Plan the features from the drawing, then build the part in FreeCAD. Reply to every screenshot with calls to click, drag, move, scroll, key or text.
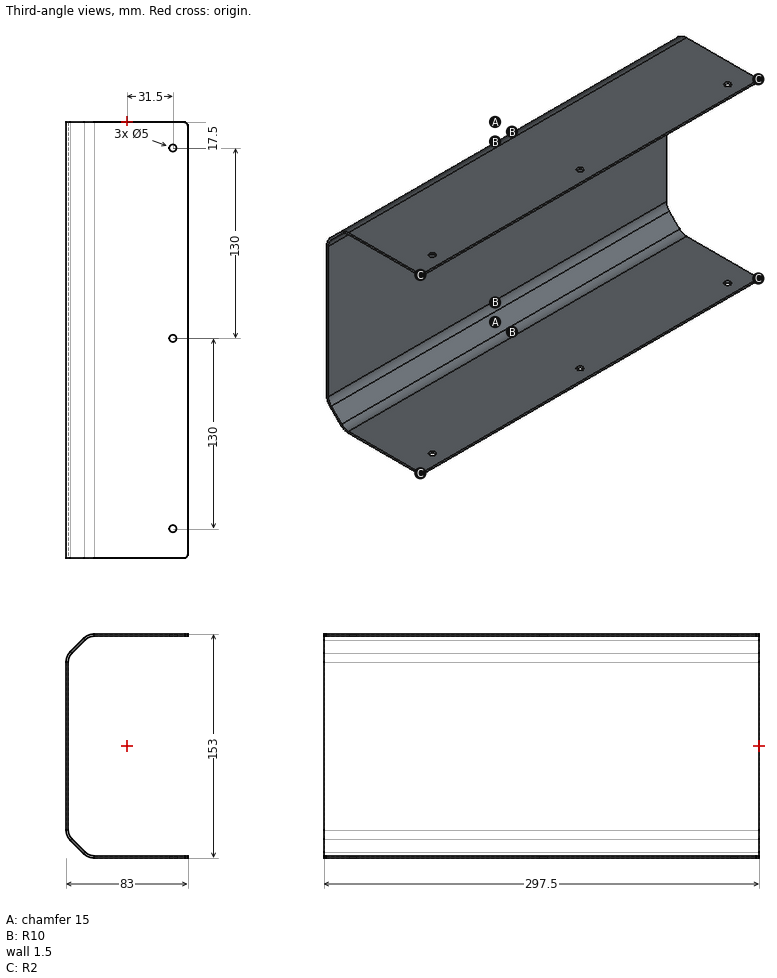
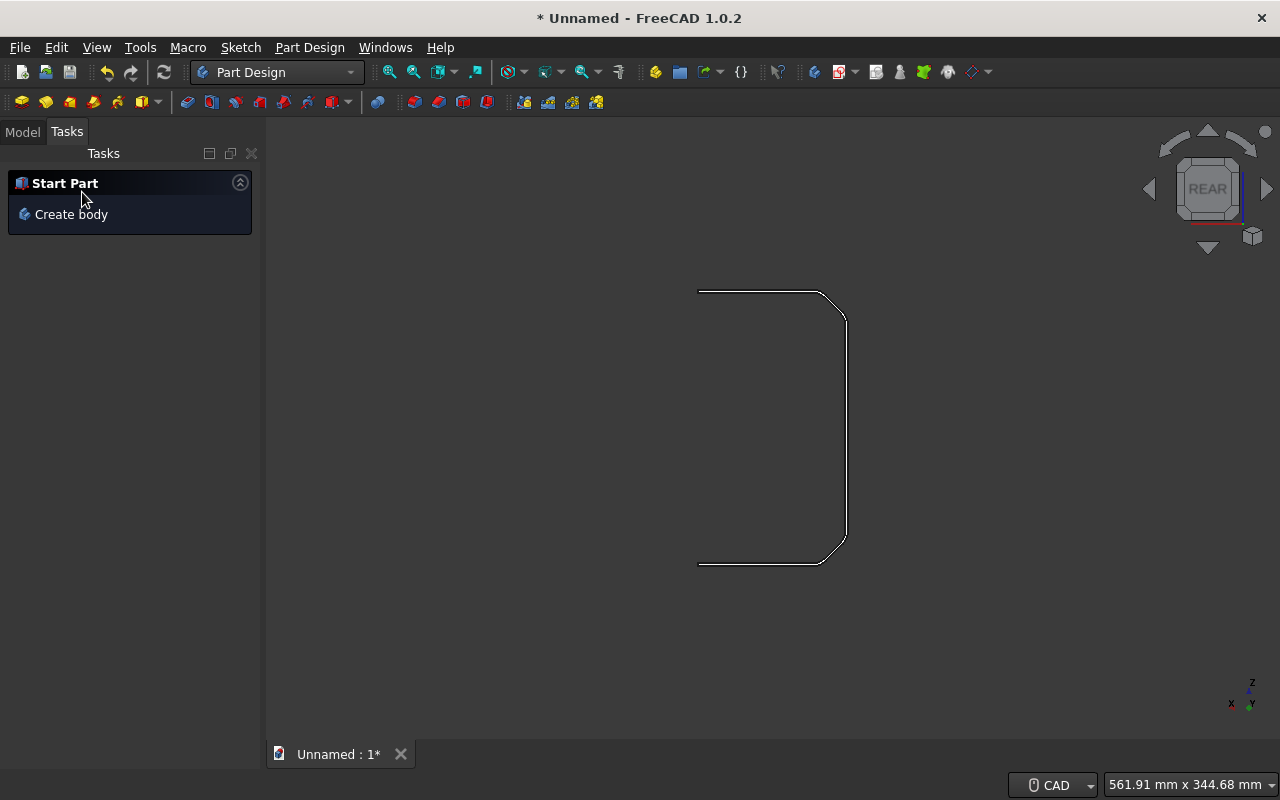
click(390, 72)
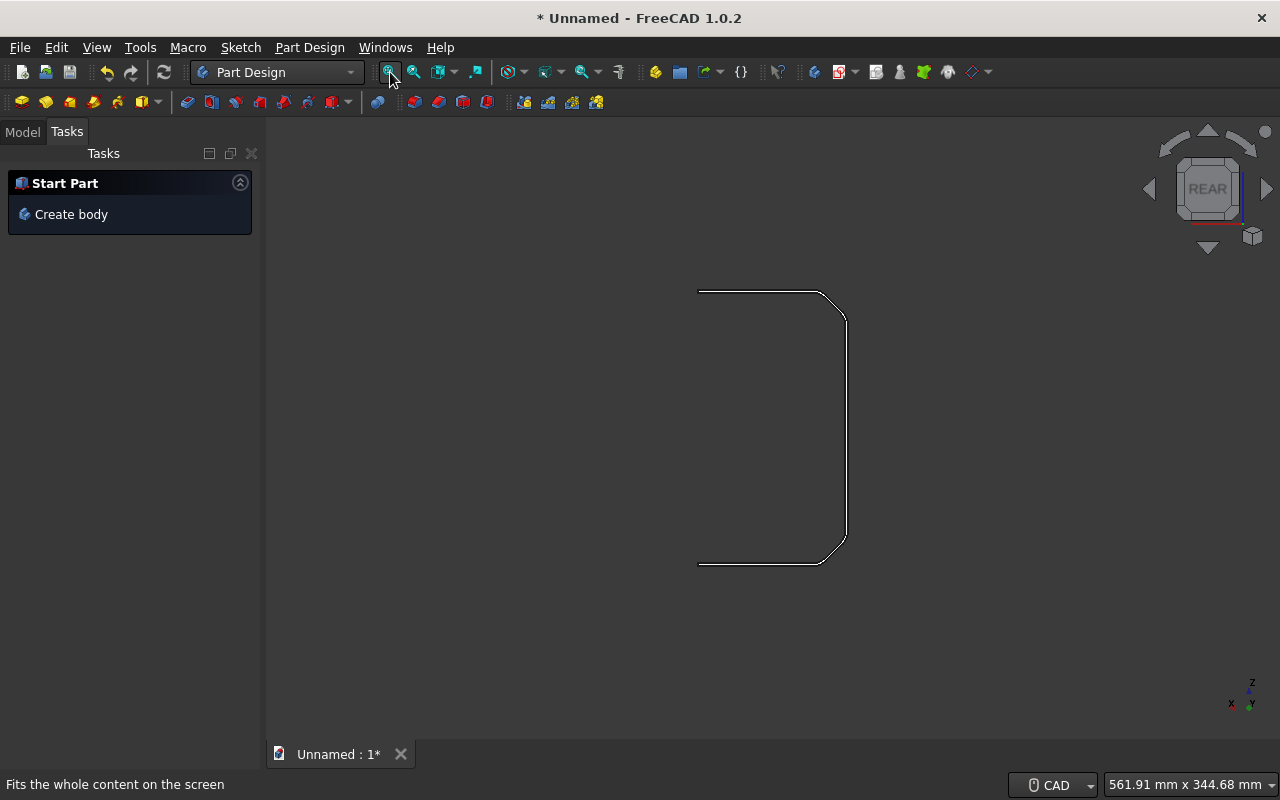
key(0)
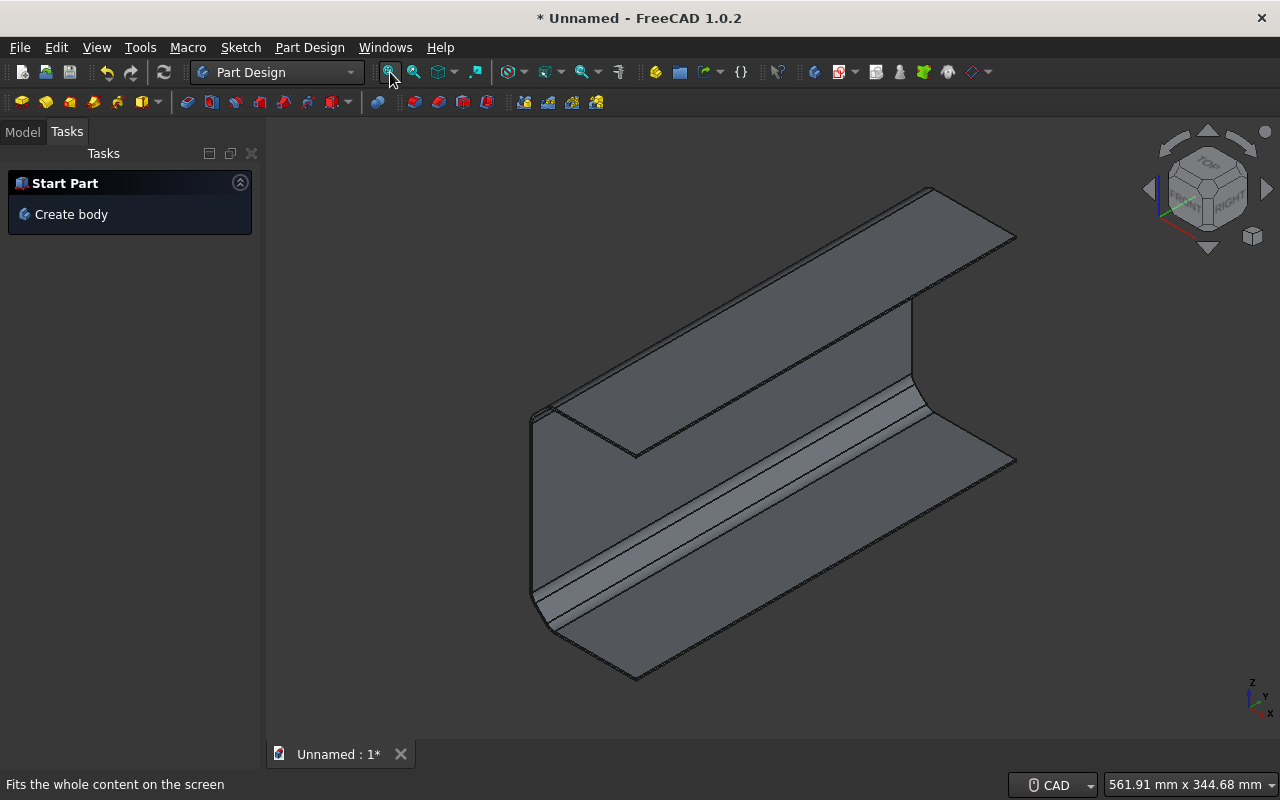
click(894, 259)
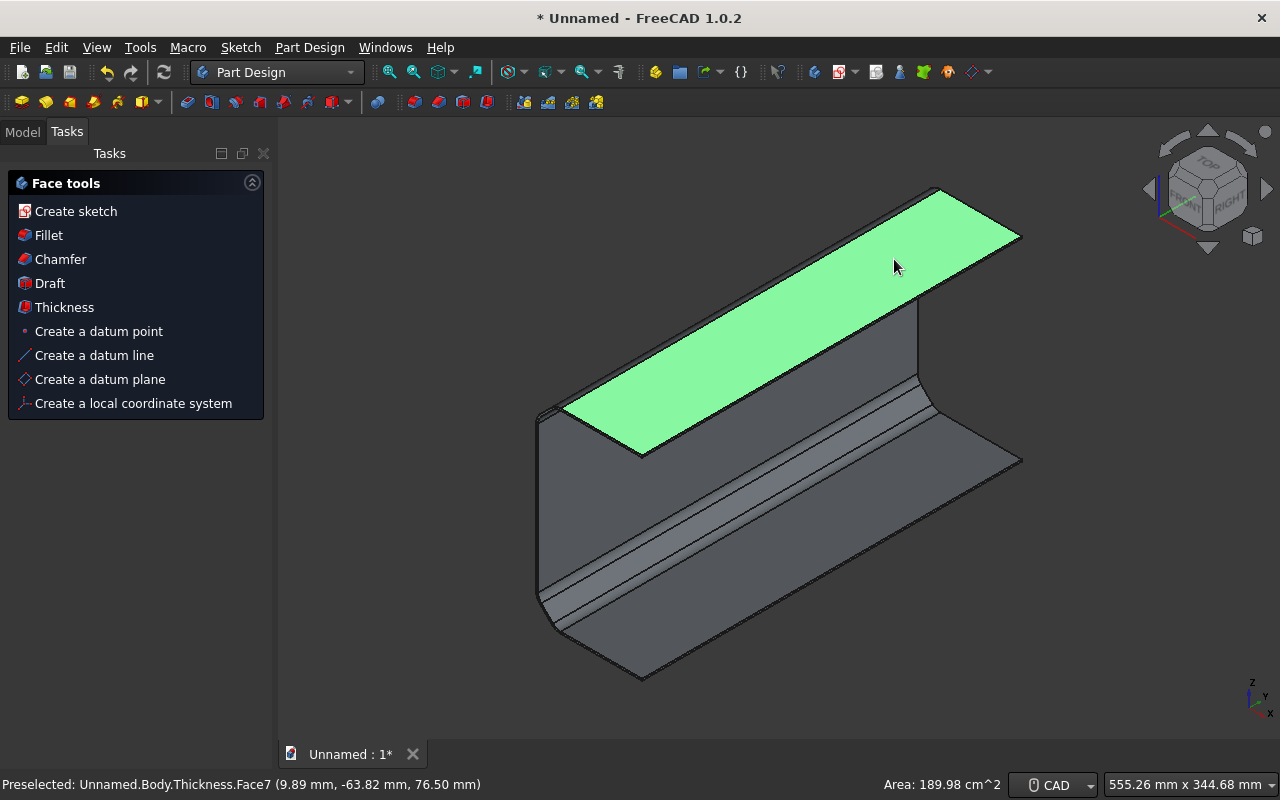
click(840, 72)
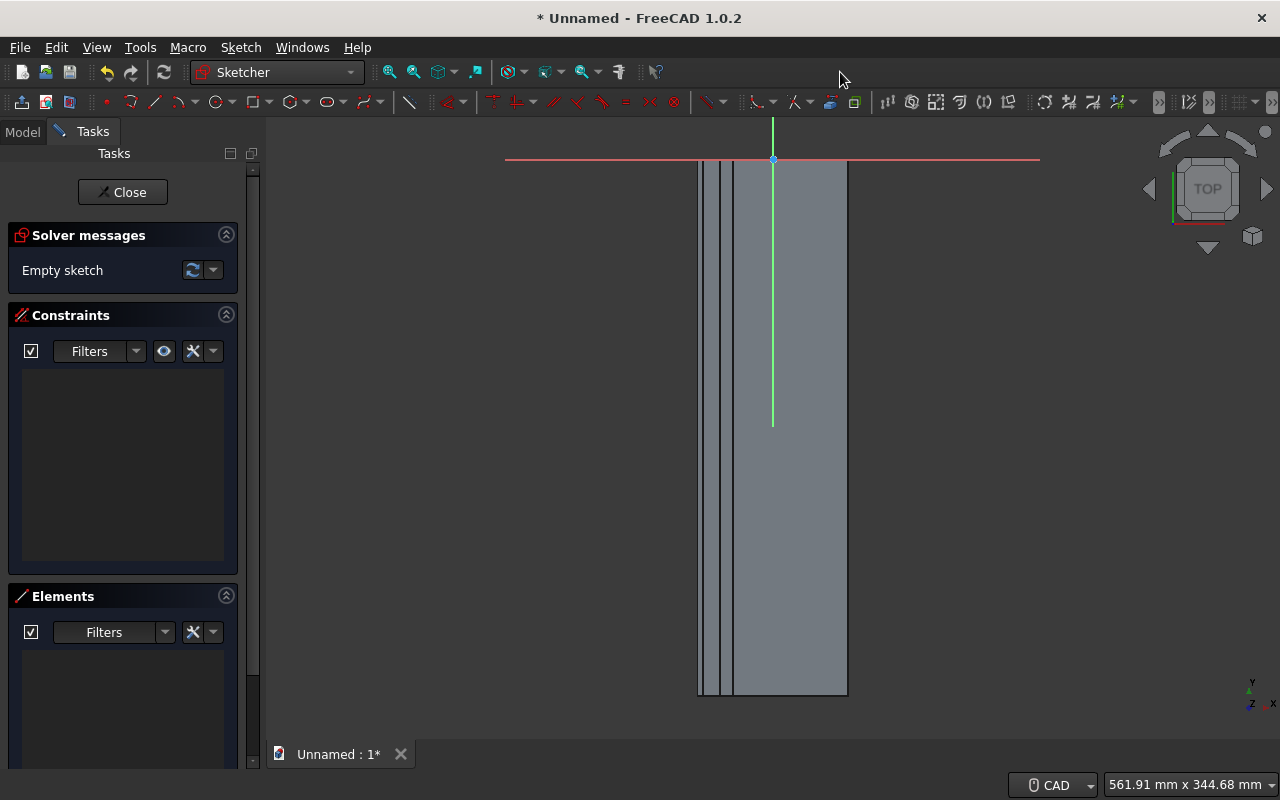
scroll(294, 499, down, 1)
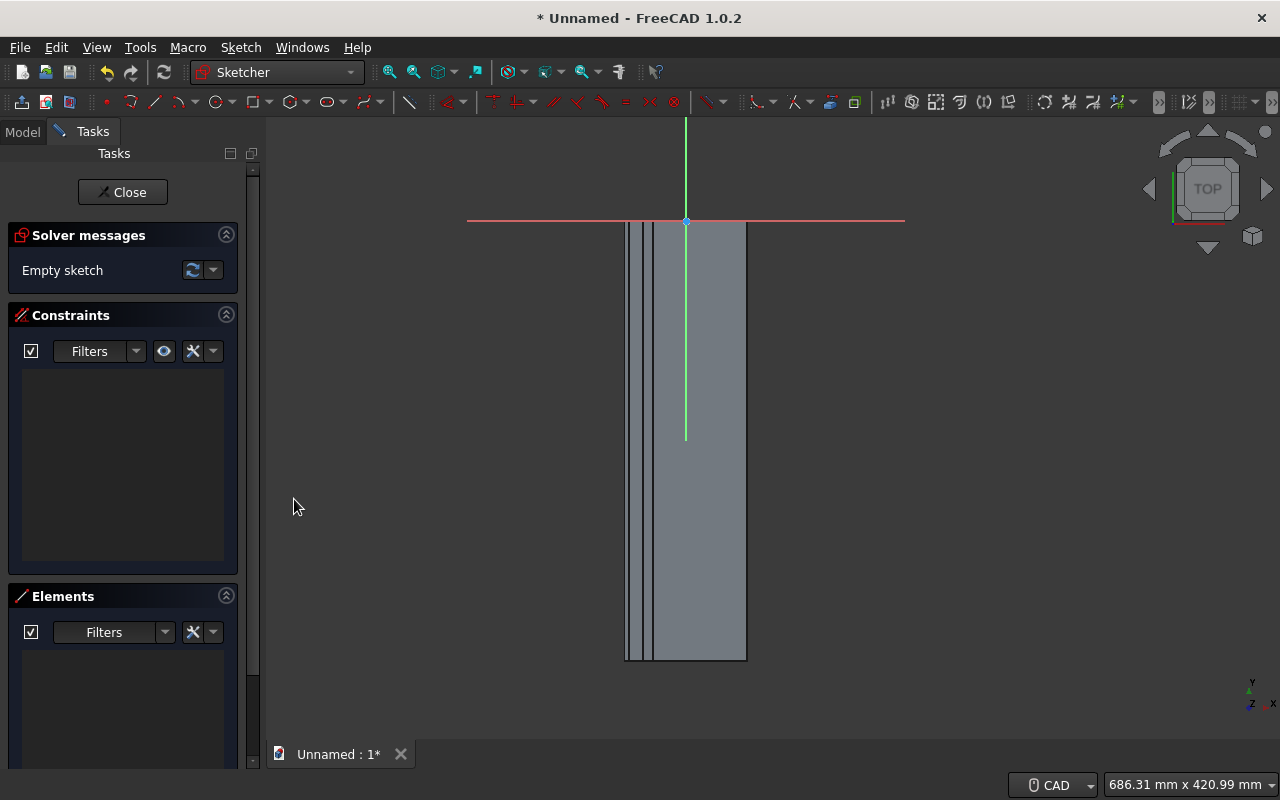
click(216, 102)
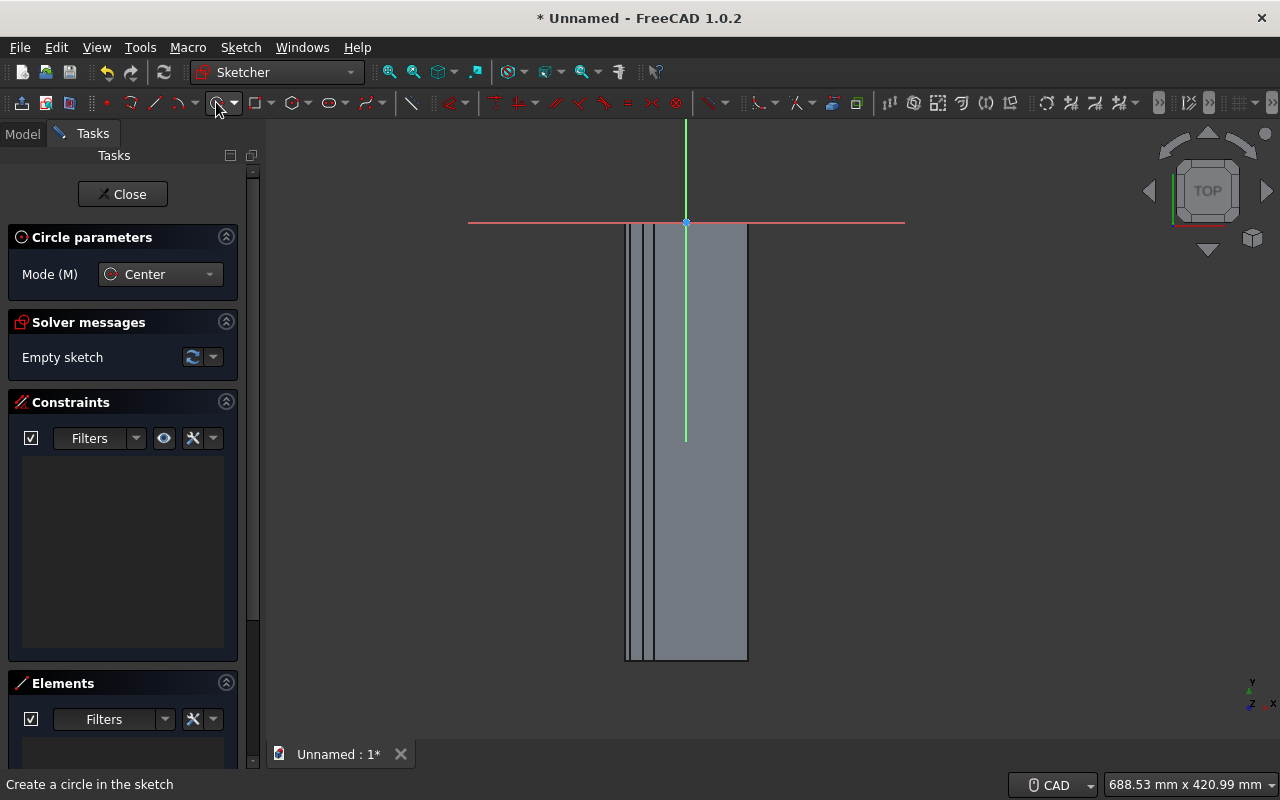
scroll(733, 249, up, 10)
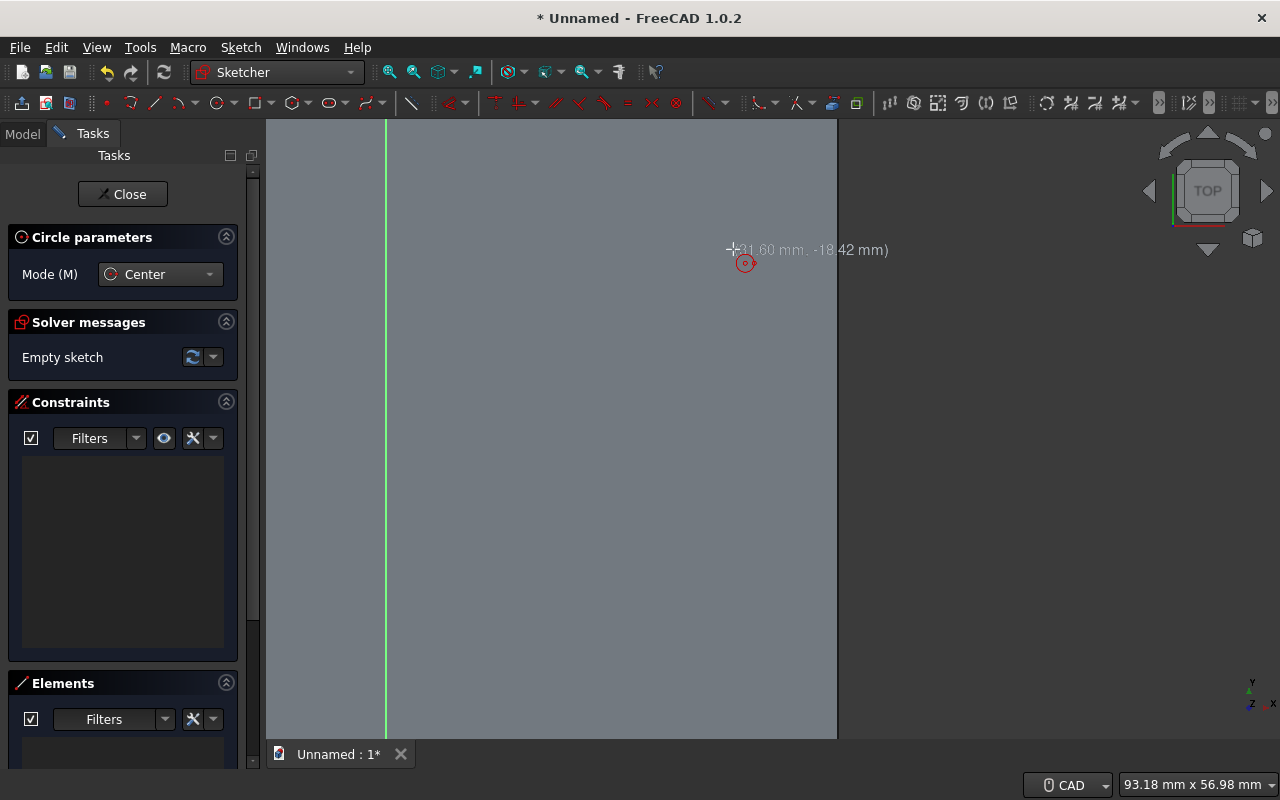
scroll(725, 249, down, 10)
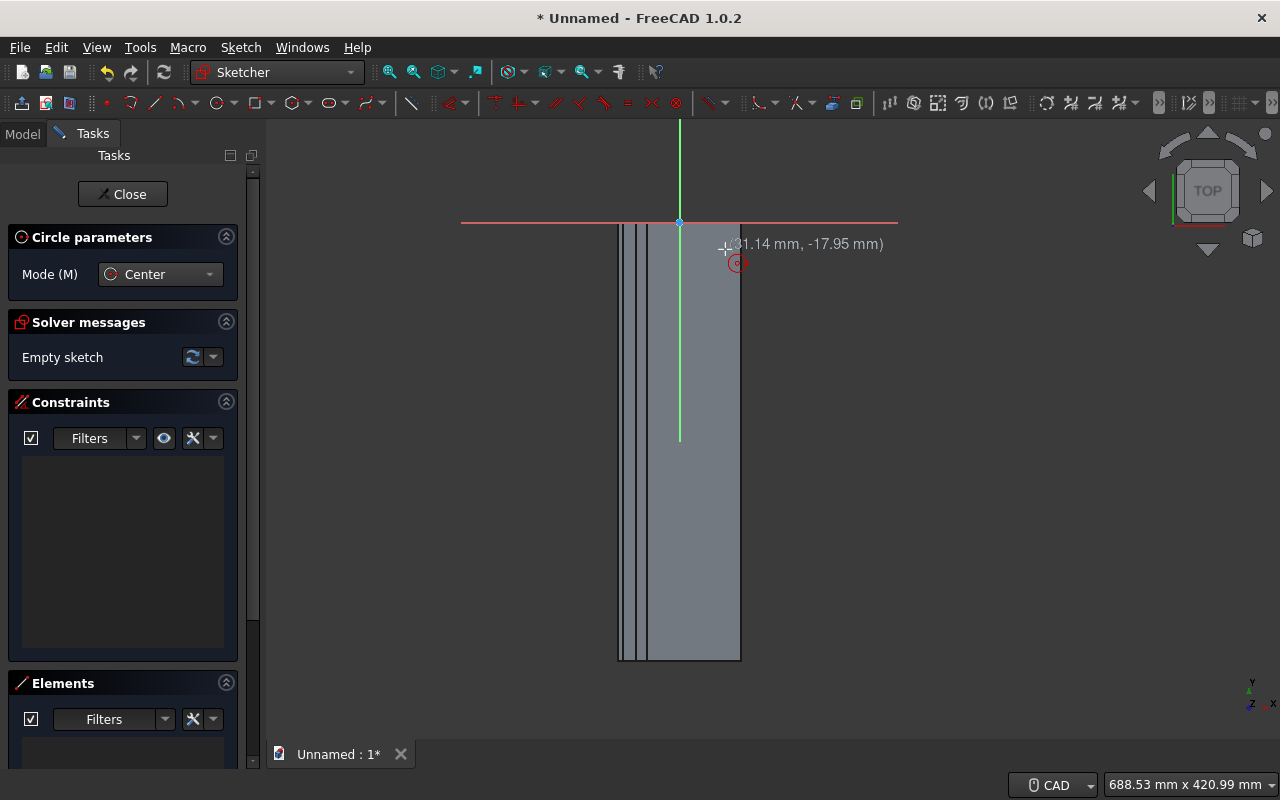
click(726, 249)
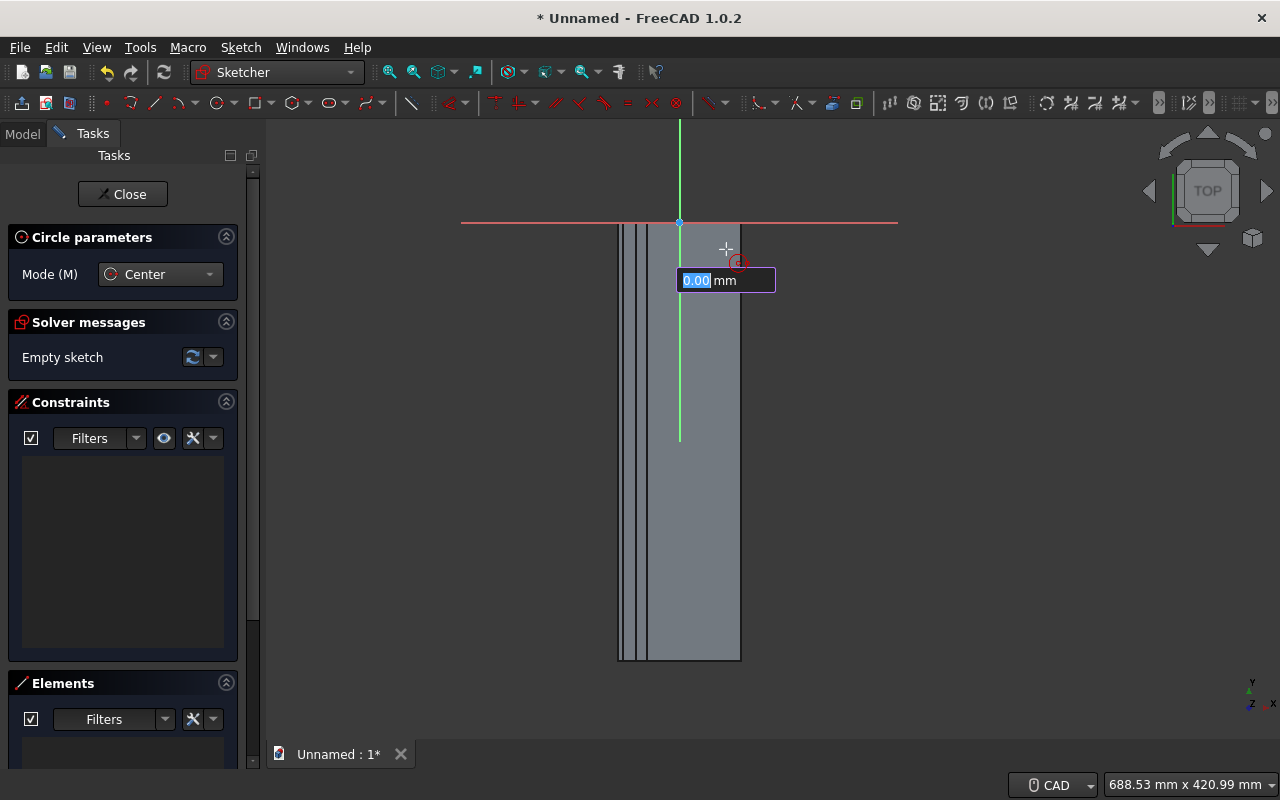
scroll(729, 246, up, 8)